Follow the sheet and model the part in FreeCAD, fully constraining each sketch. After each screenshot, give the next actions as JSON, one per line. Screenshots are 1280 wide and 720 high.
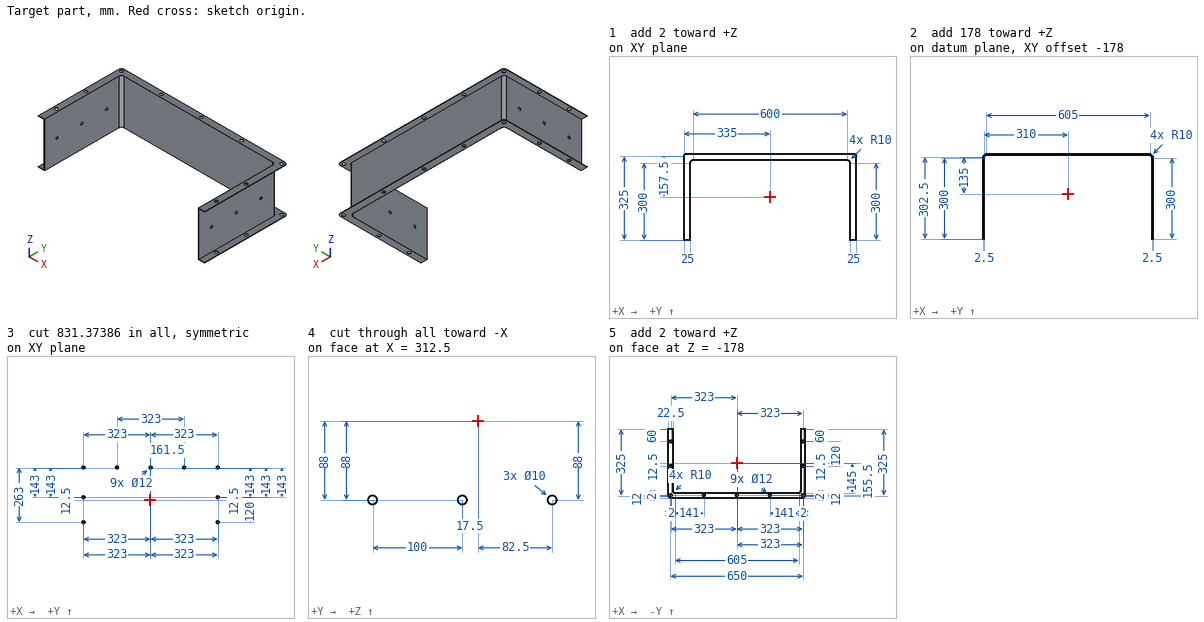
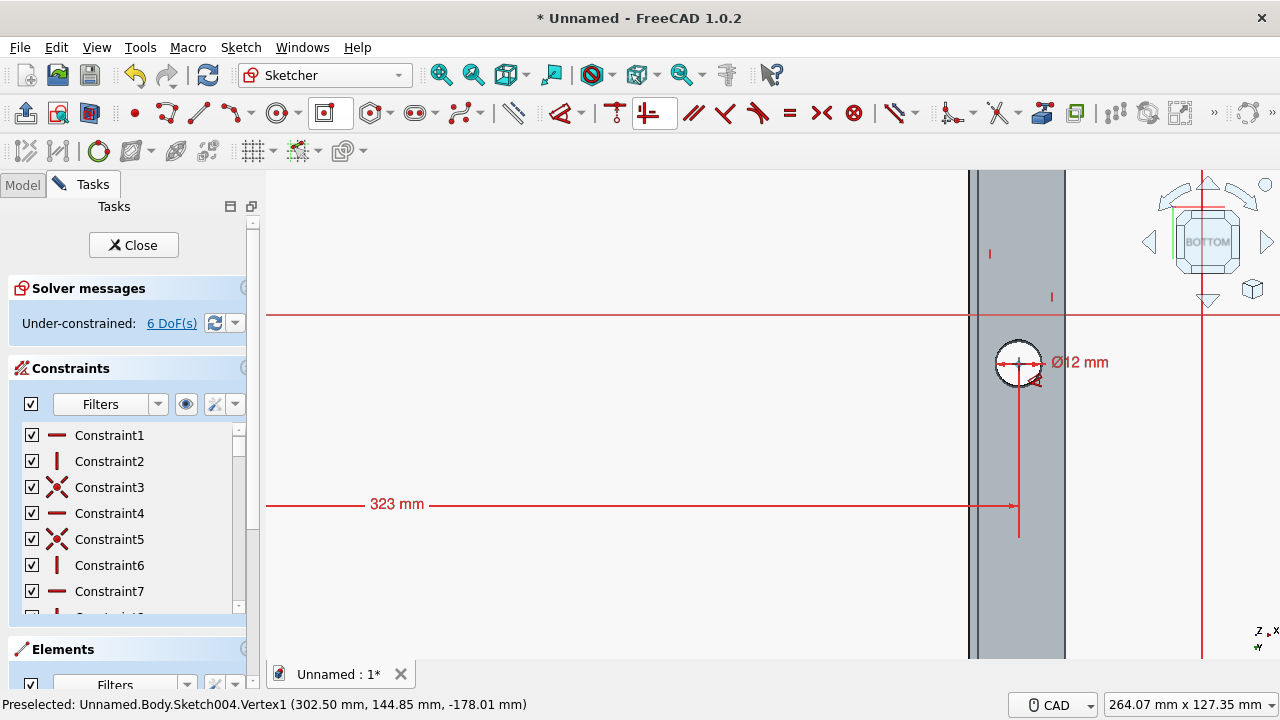
{"action": "left_click", "coordinate": [1019, 364]}
{"action": "left_click", "coordinate": [1101, 340]}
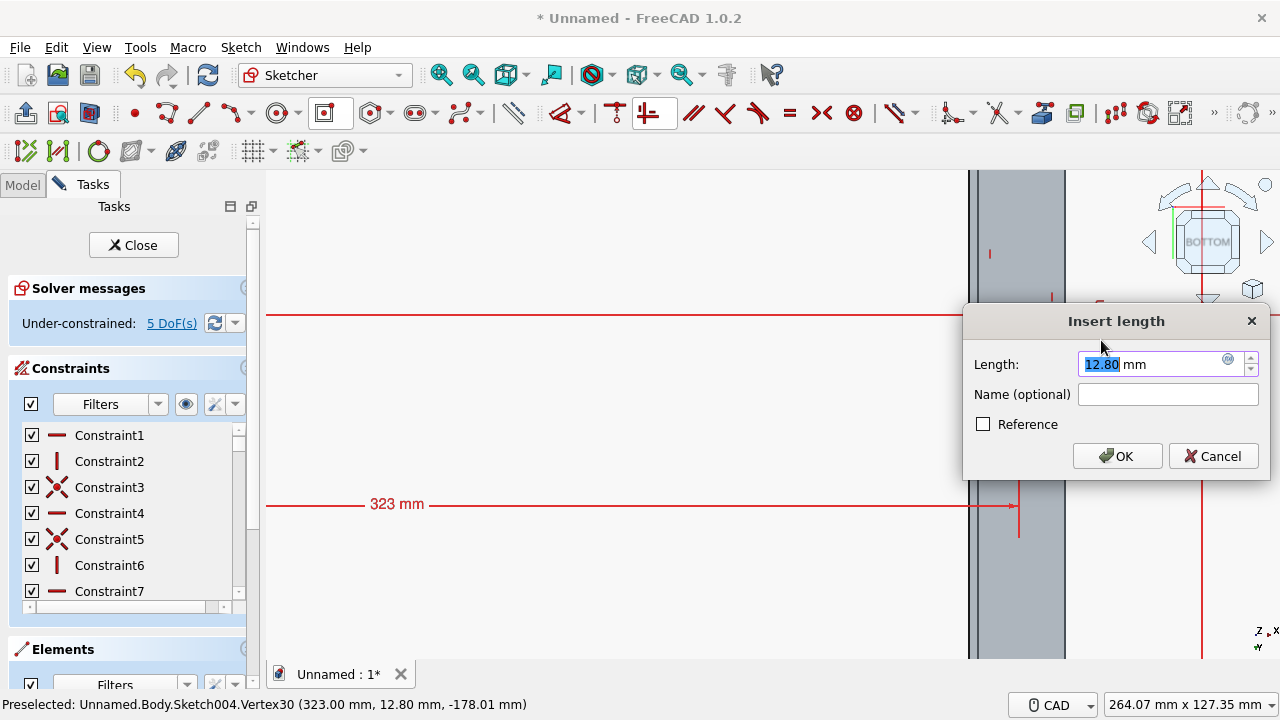
{"action": "type", "text": "12.5"}
{"action": "key", "text": "Return"}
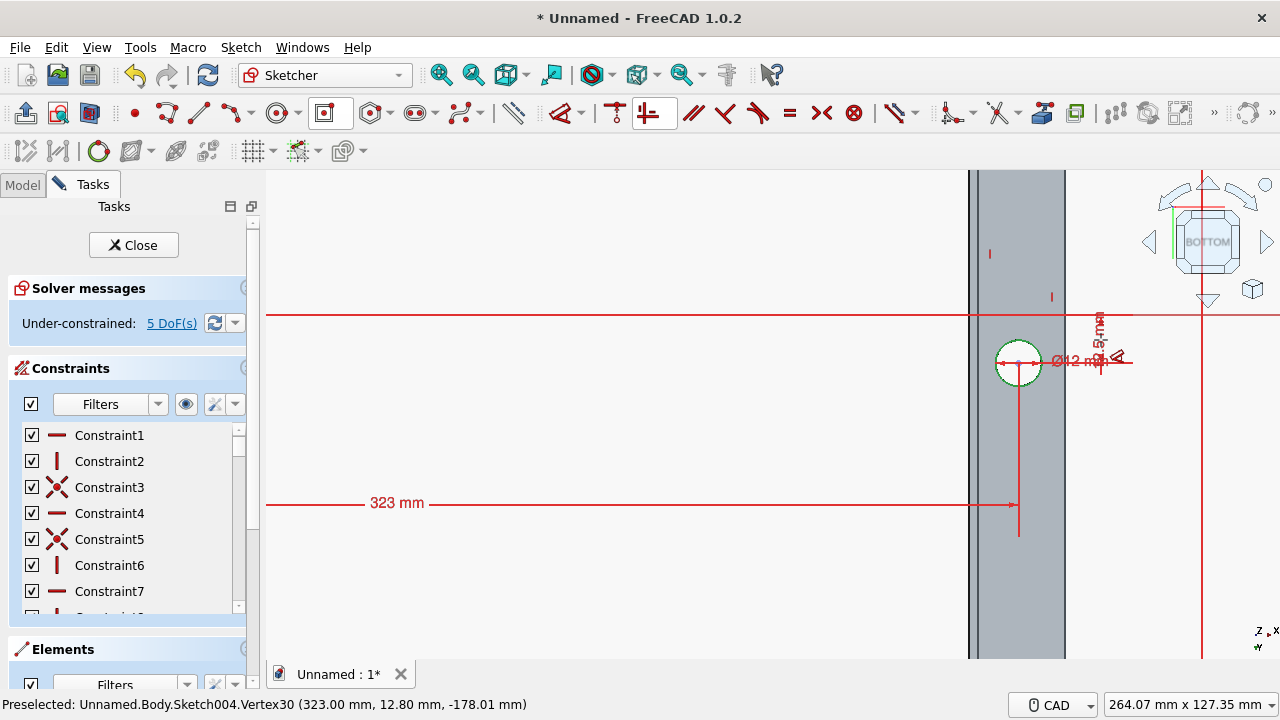
{"action": "scroll", "coordinate": [1008, 447], "scroll_direction": "down", "scroll_amount": 7}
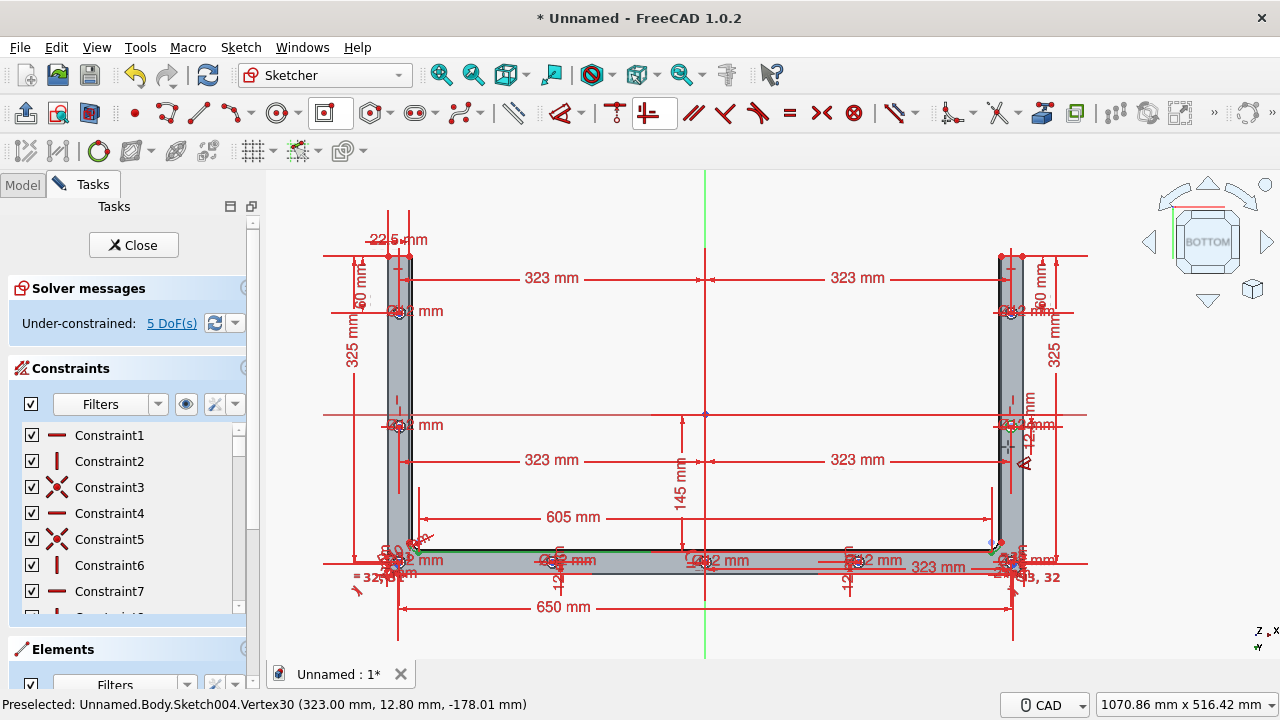
{"action": "scroll", "coordinate": [399, 427], "scroll_direction": "up", "scroll_amount": 7}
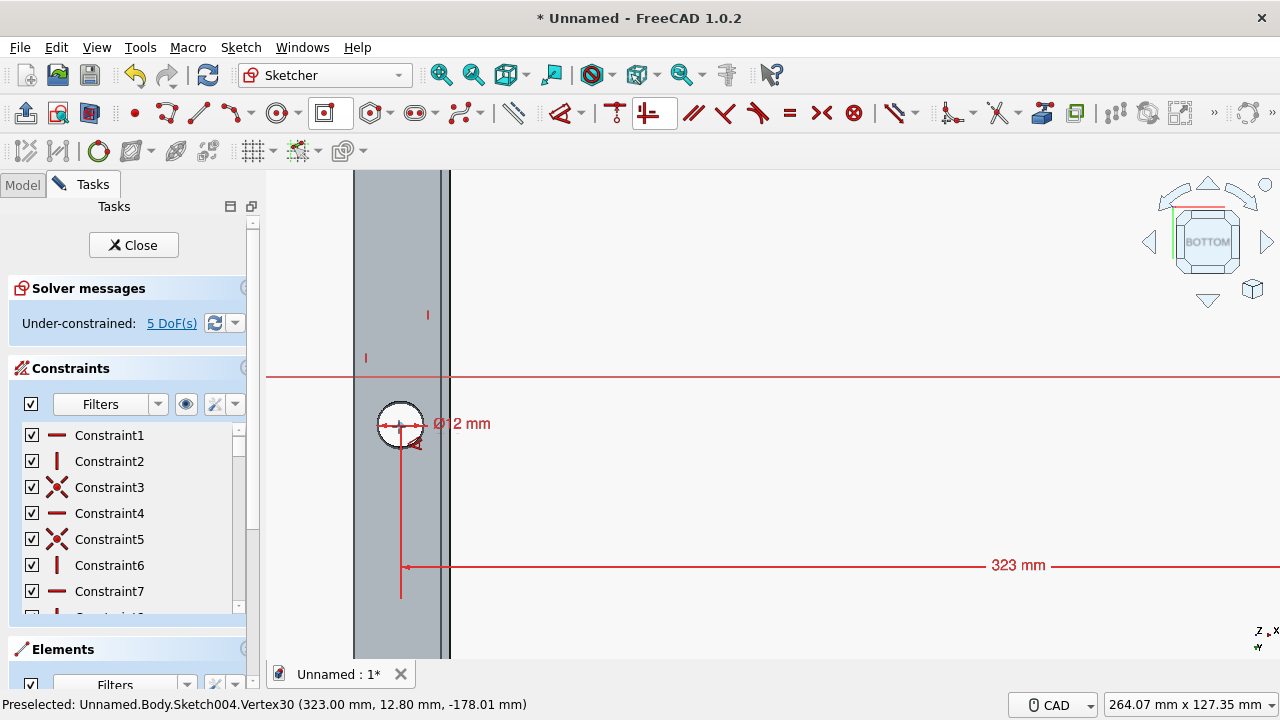
{"action": "left_click", "coordinate": [401, 426]}
{"action": "left_click", "coordinate": [319, 401]}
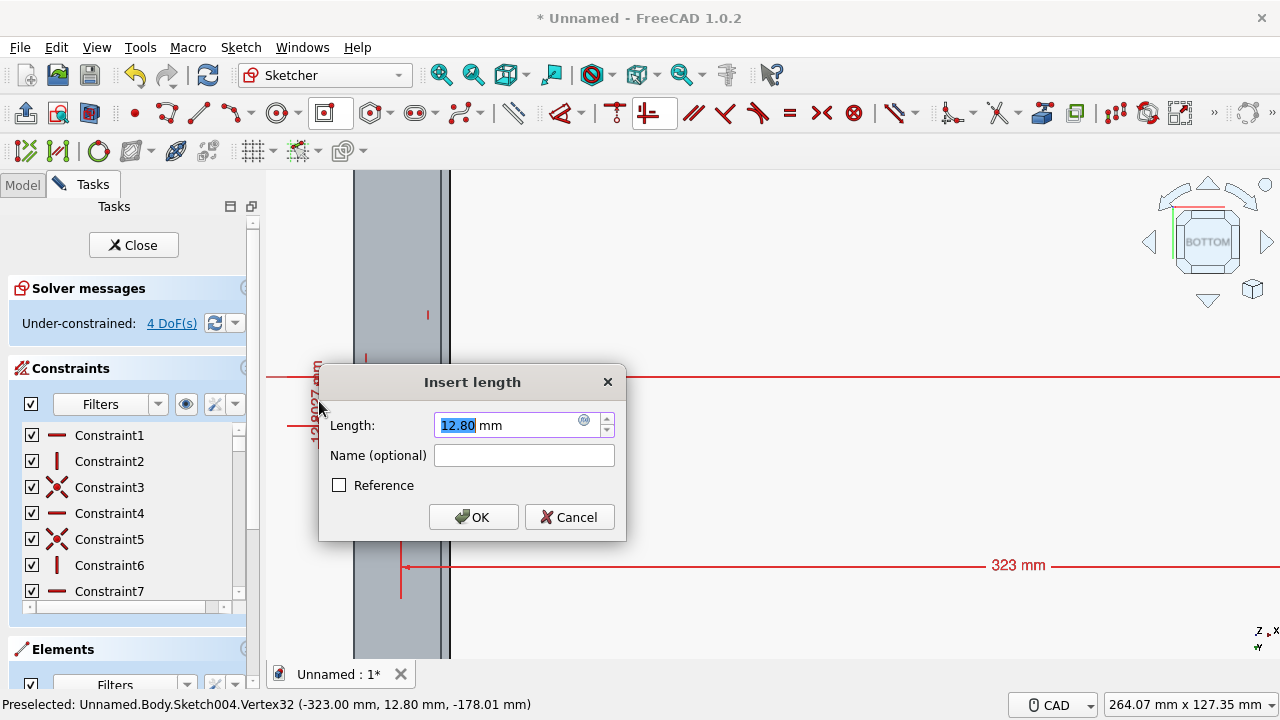
{"action": "type", "text": "12.5"}
{"action": "key", "text": "Return"}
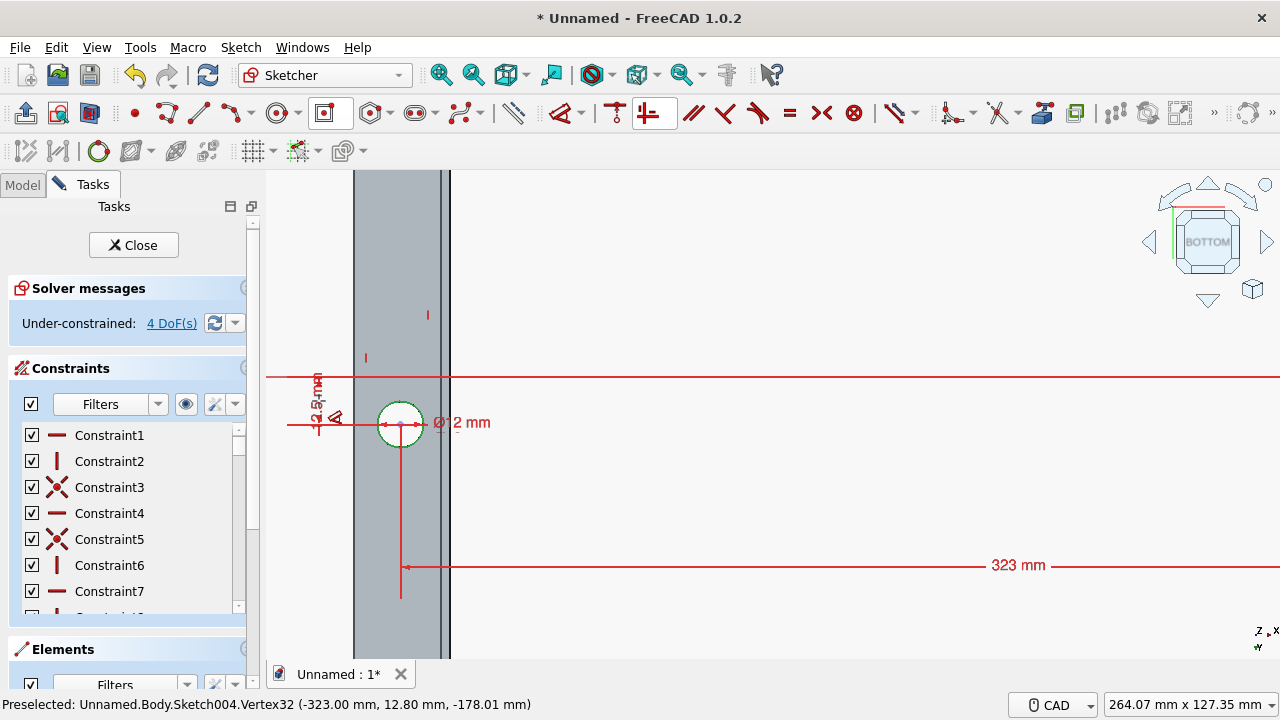
{"action": "scroll", "coordinate": [398, 427], "scroll_direction": "down", "scroll_amount": 7}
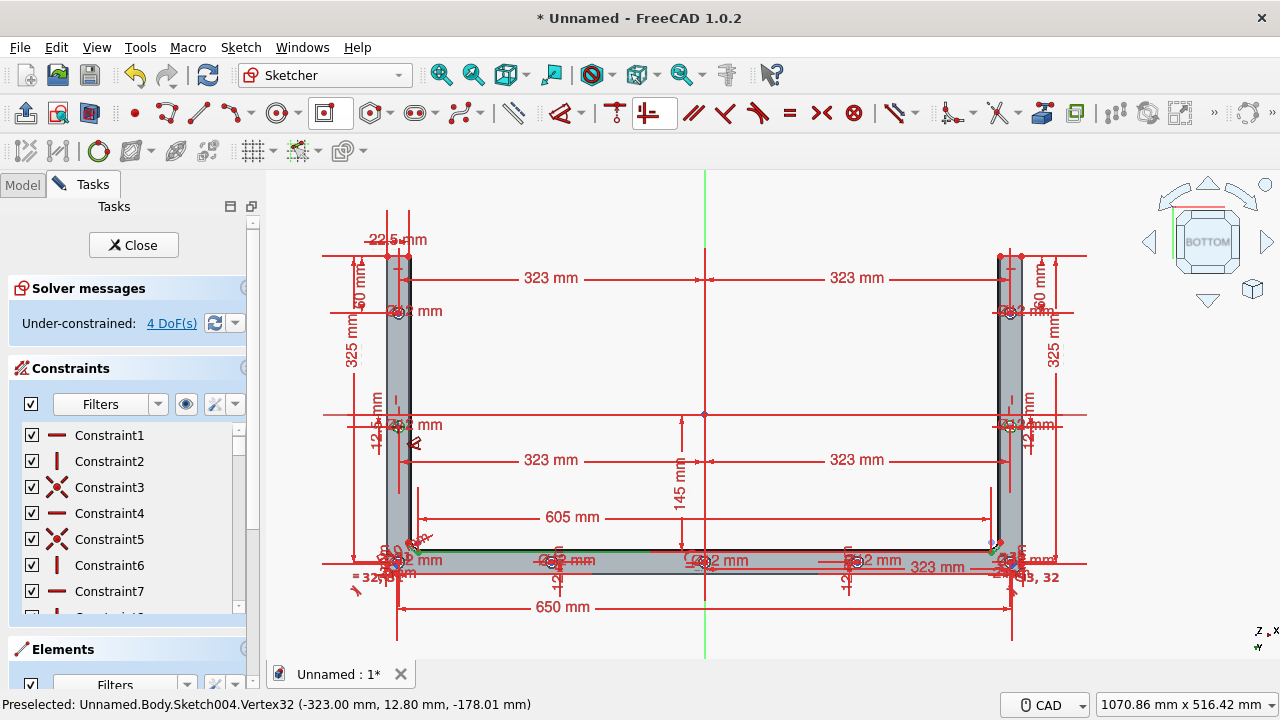
{"action": "left_click", "coordinate": [1010, 313]}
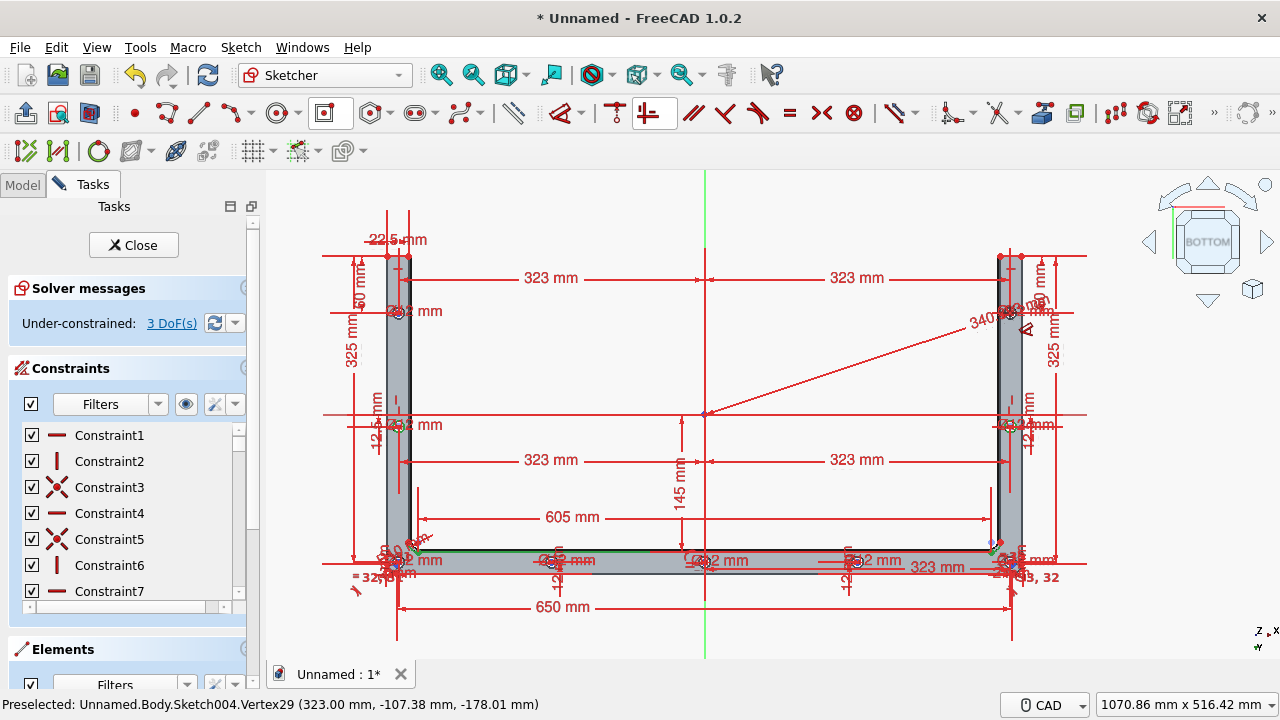
{"action": "left_click", "coordinate": [1010, 427]}
{"action": "left_click", "coordinate": [1044, 370]}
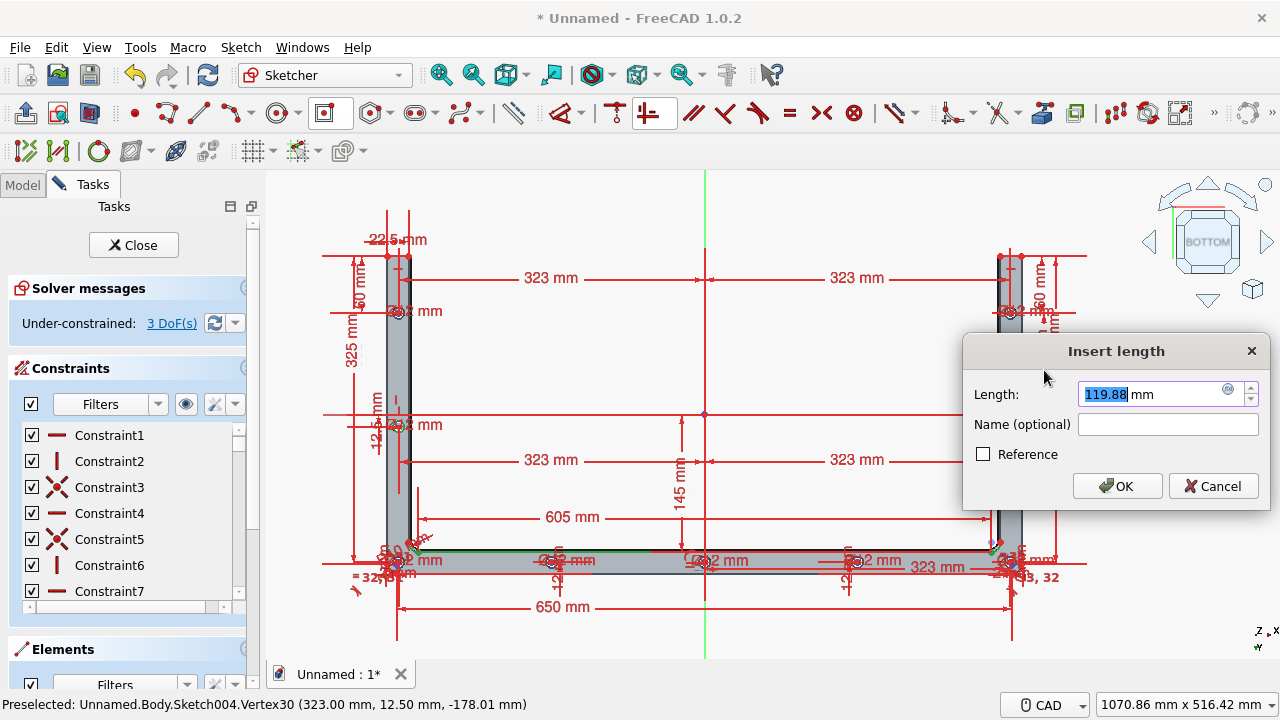
{"action": "type", "text": "120"}
{"action": "key", "text": "Return"}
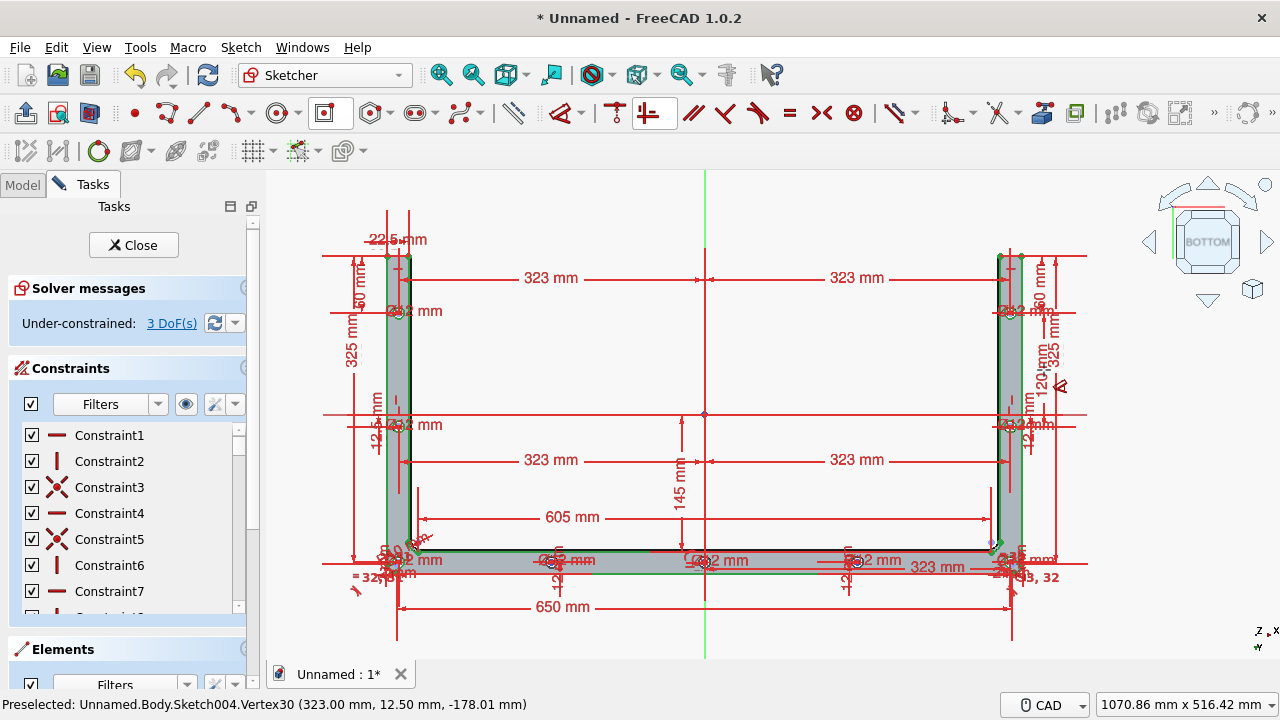
{"action": "scroll", "coordinate": [991, 552], "scroll_direction": "up", "scroll_amount": 2}